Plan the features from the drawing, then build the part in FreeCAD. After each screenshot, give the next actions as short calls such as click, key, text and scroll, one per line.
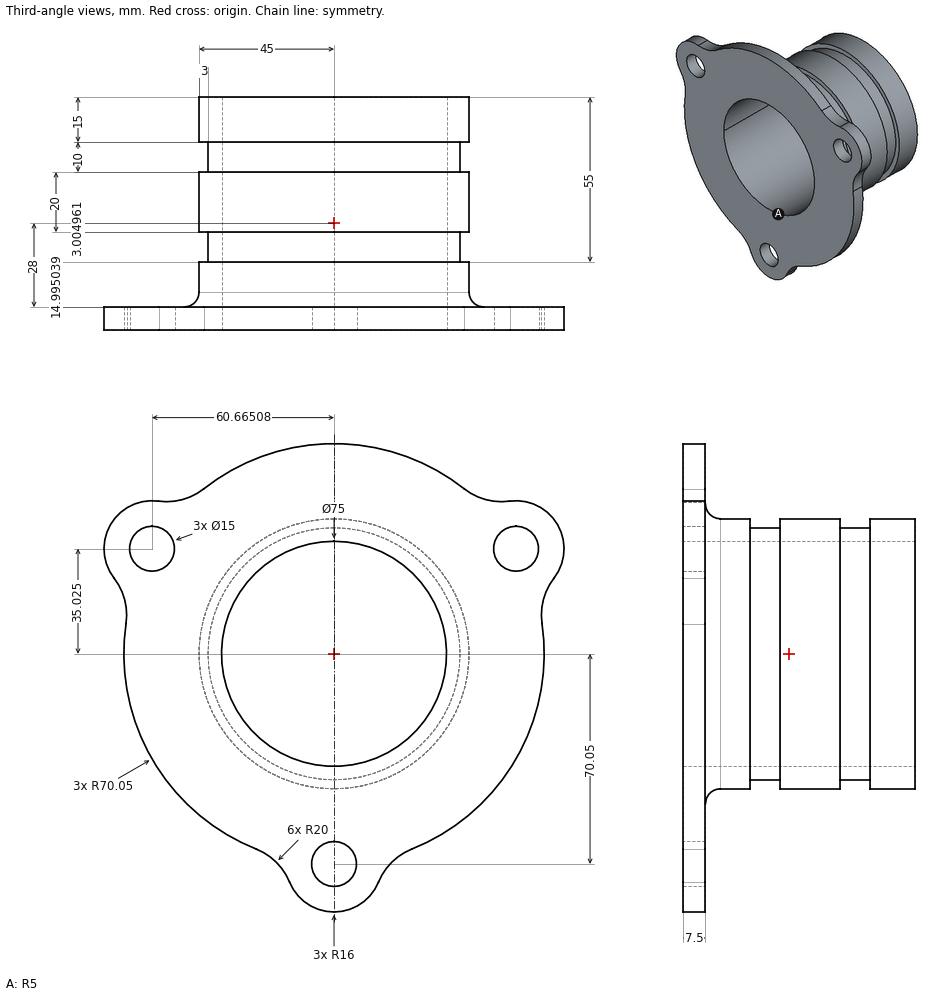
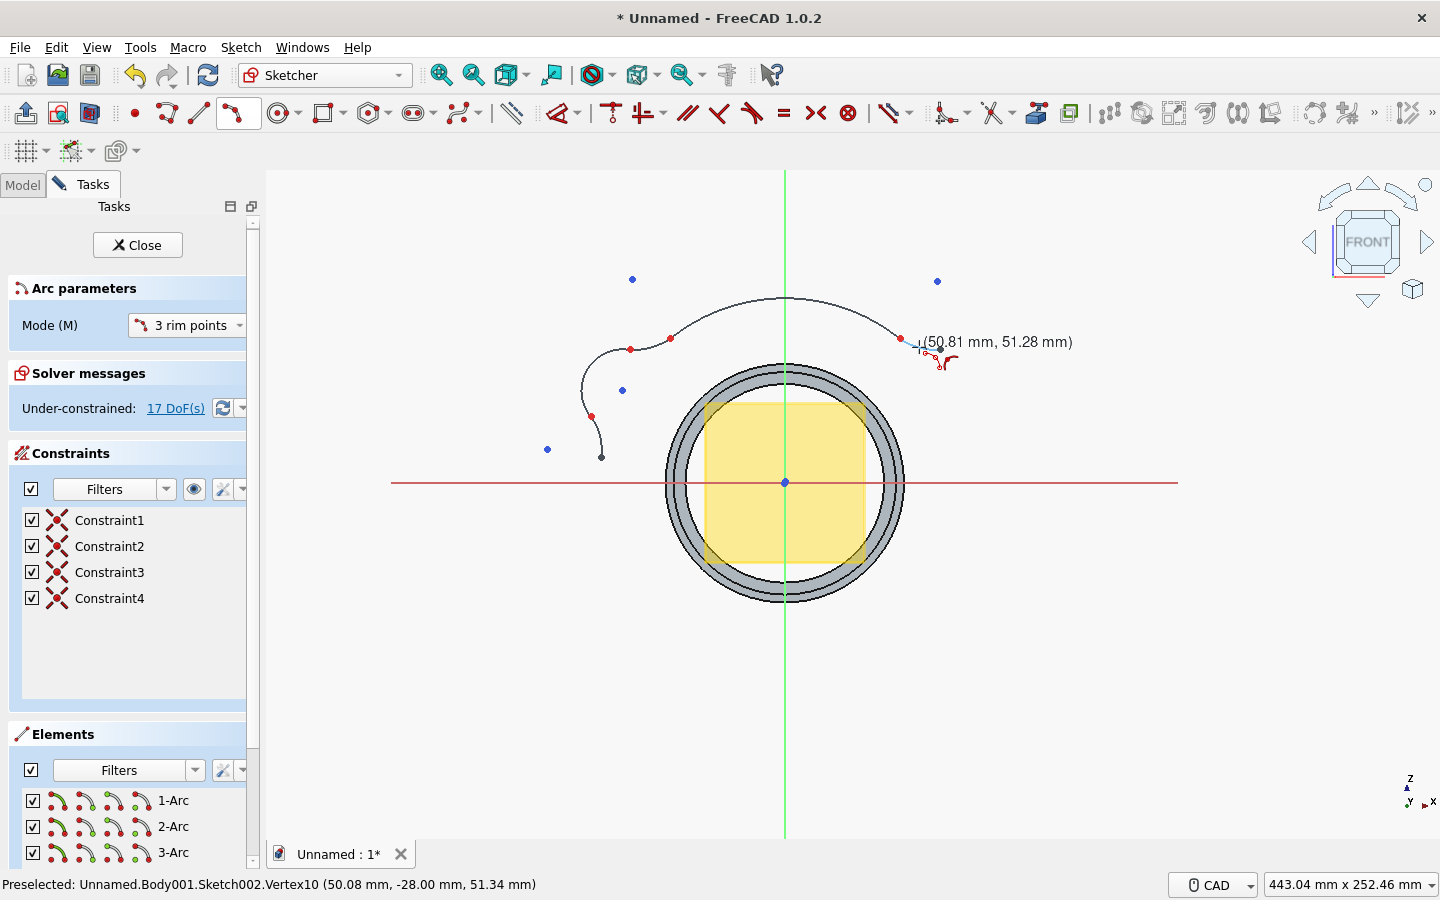
click(940, 350)
click(979, 416)
click(982, 369)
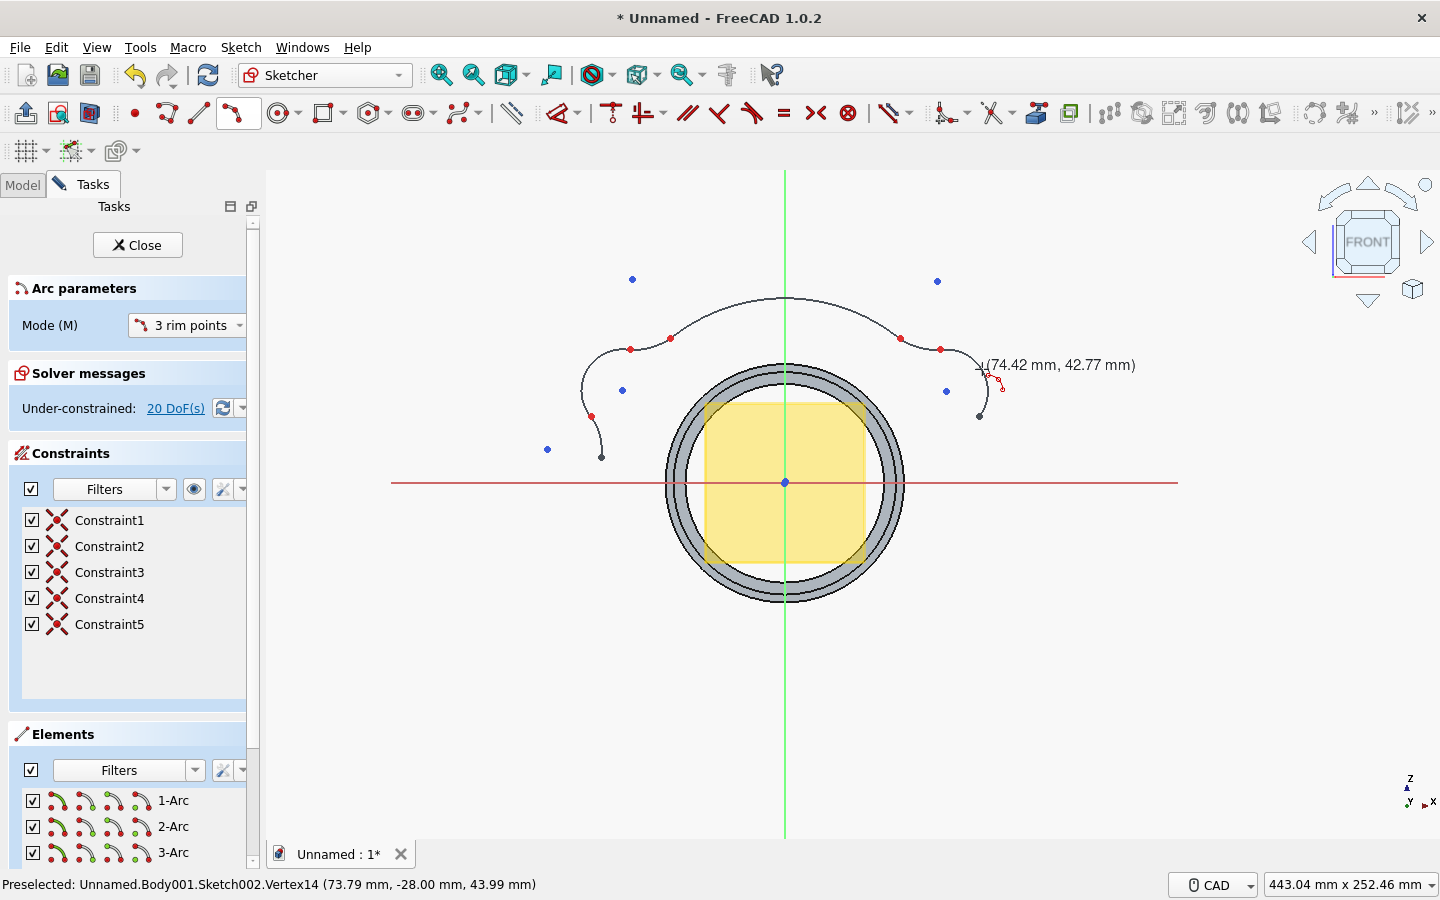
click(979, 417)
click(968, 457)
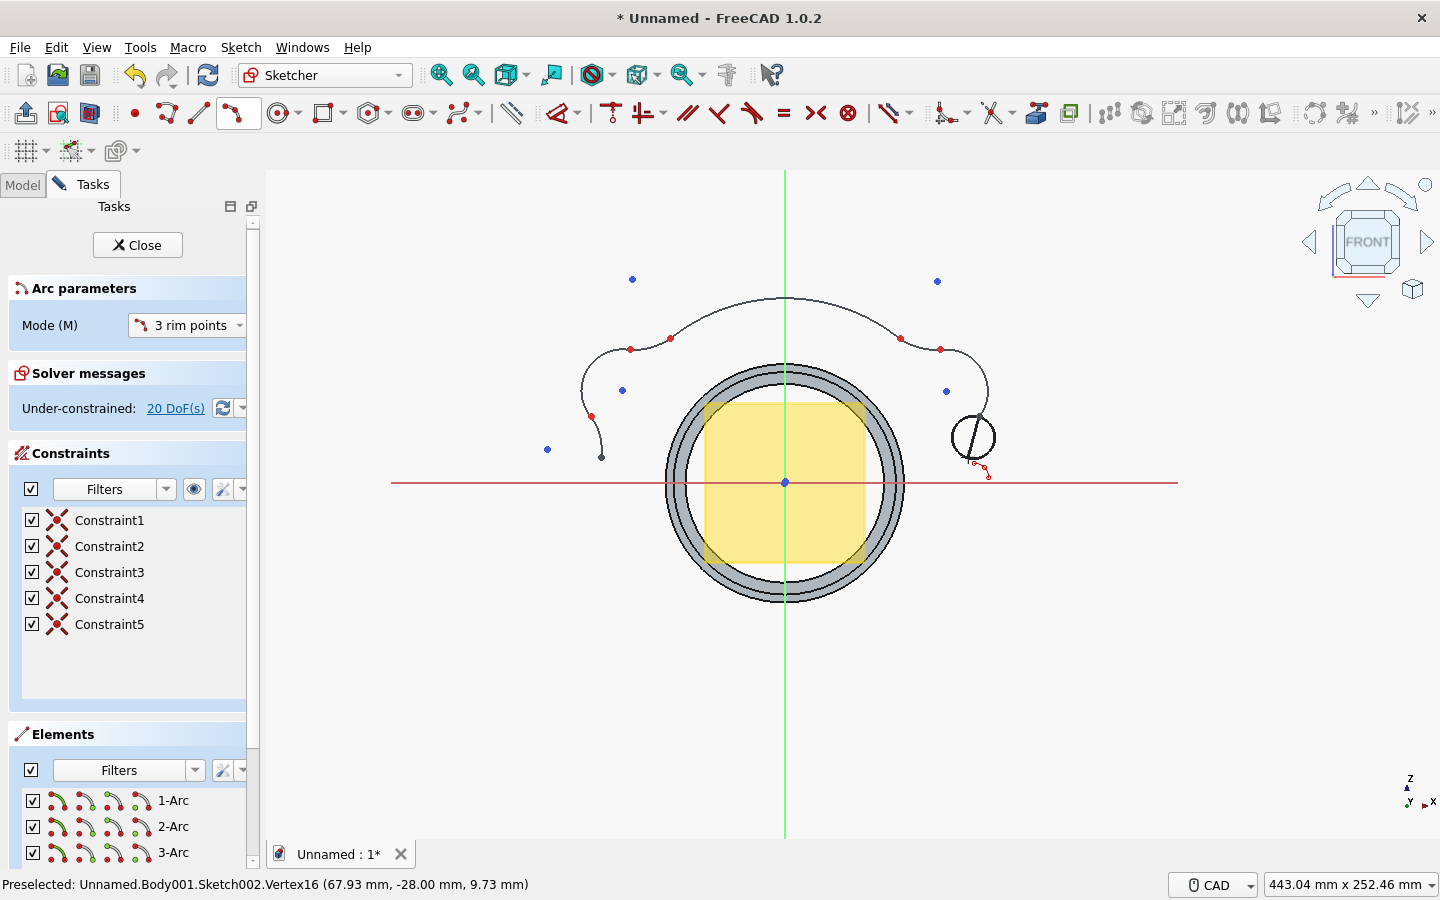
scroll(970, 435, up, 7)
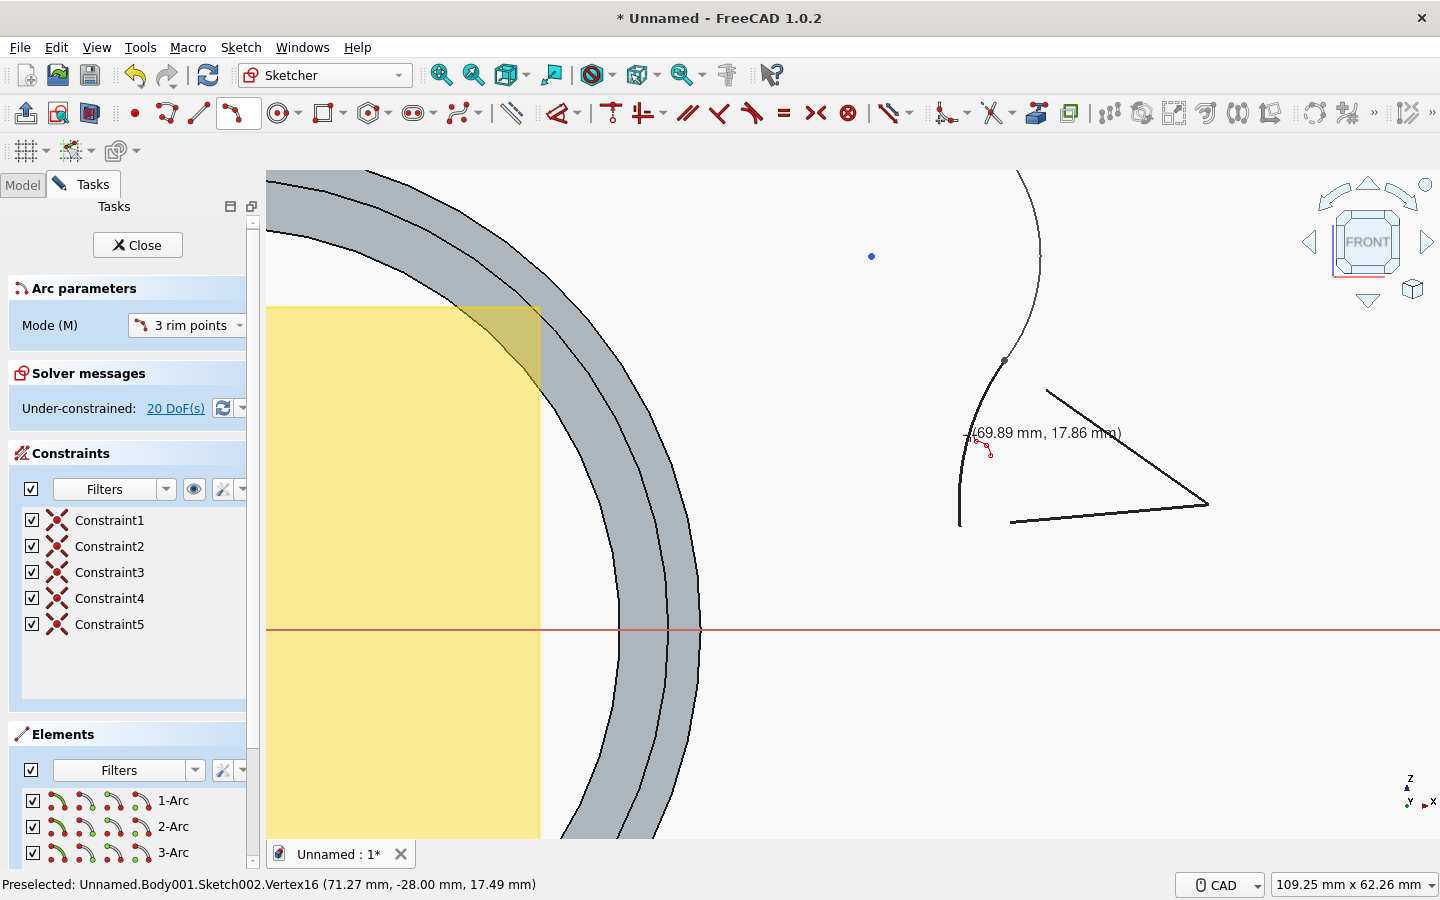
click(967, 436)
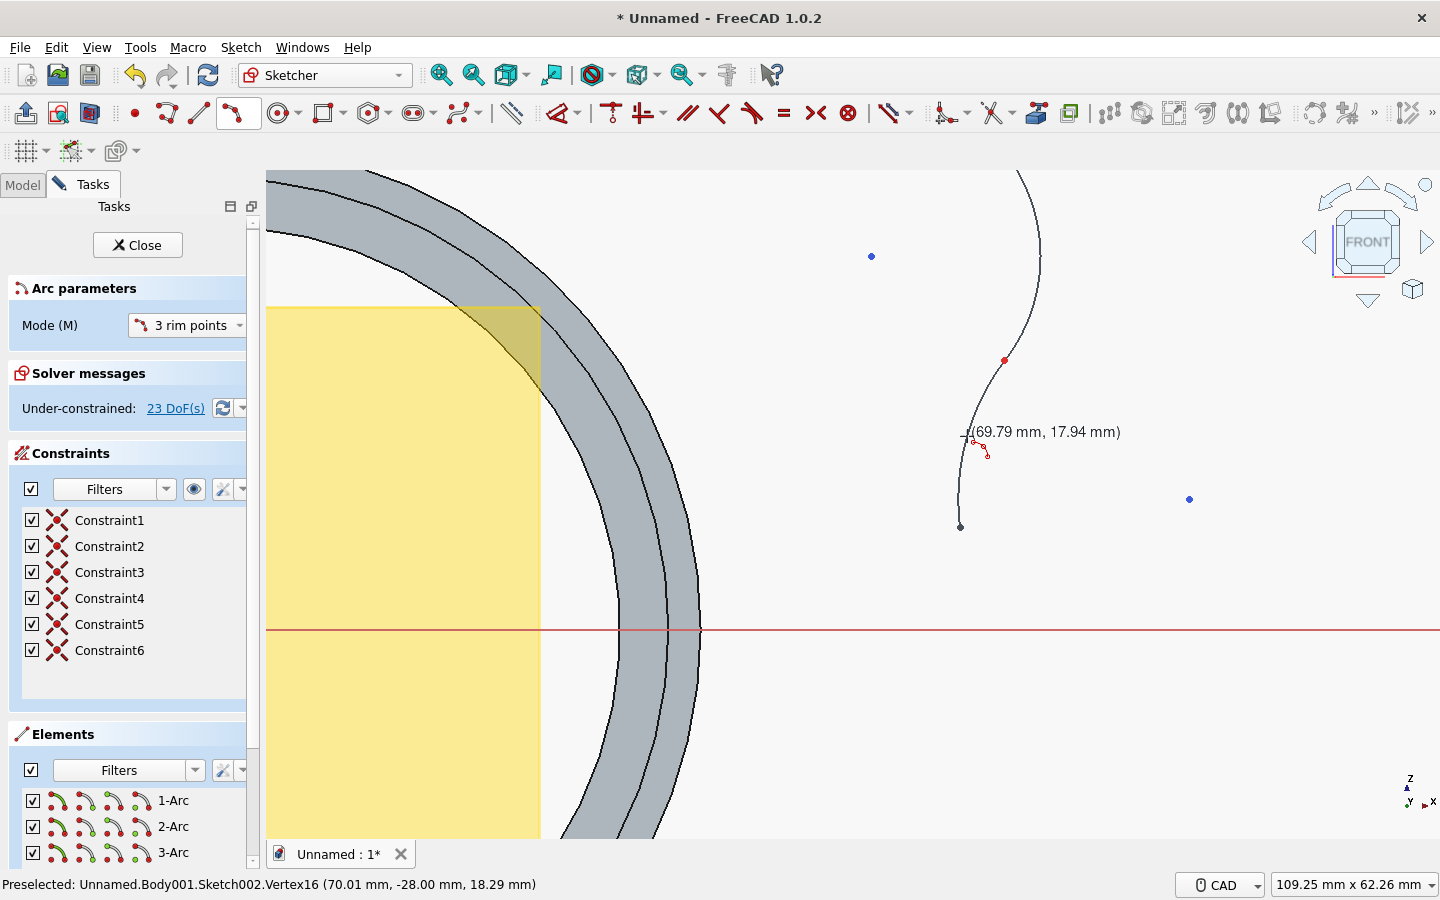
scroll(970, 435, down, 7)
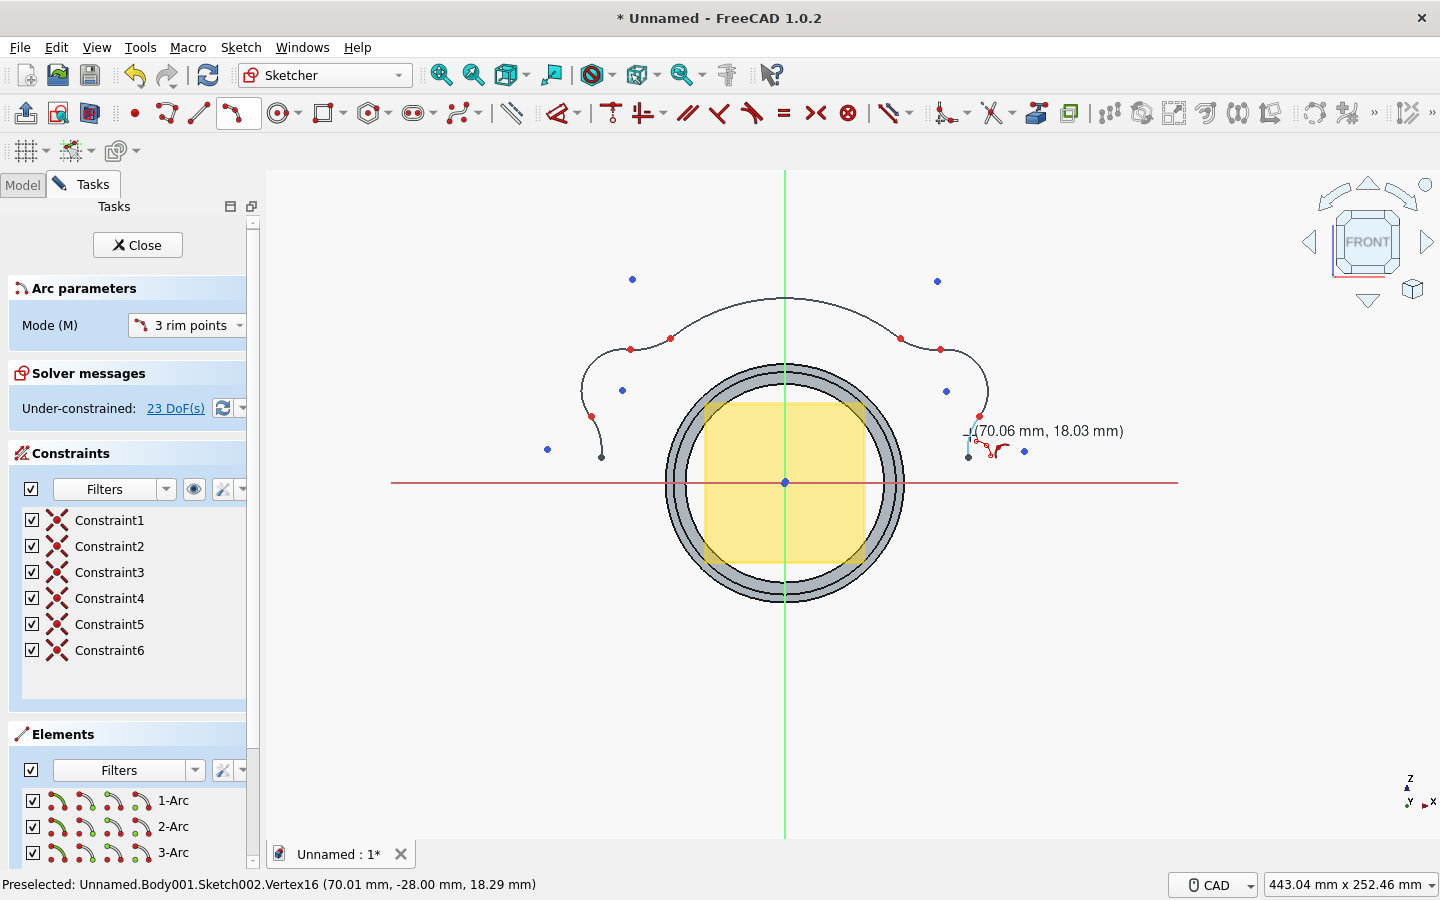
click(968, 458)
click(853, 656)
click(946, 576)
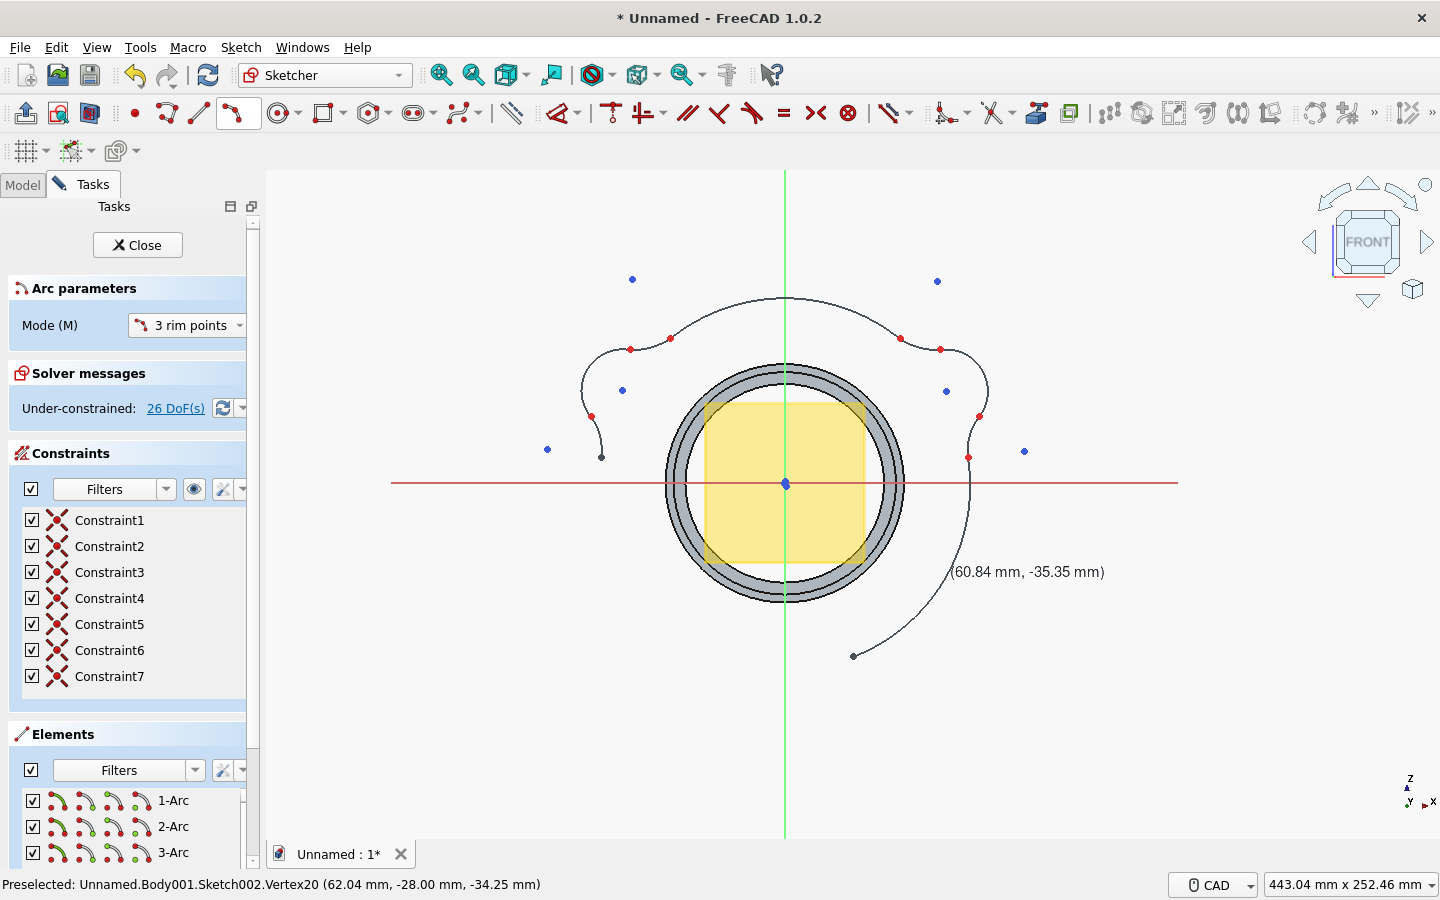
click(853, 657)
click(824, 685)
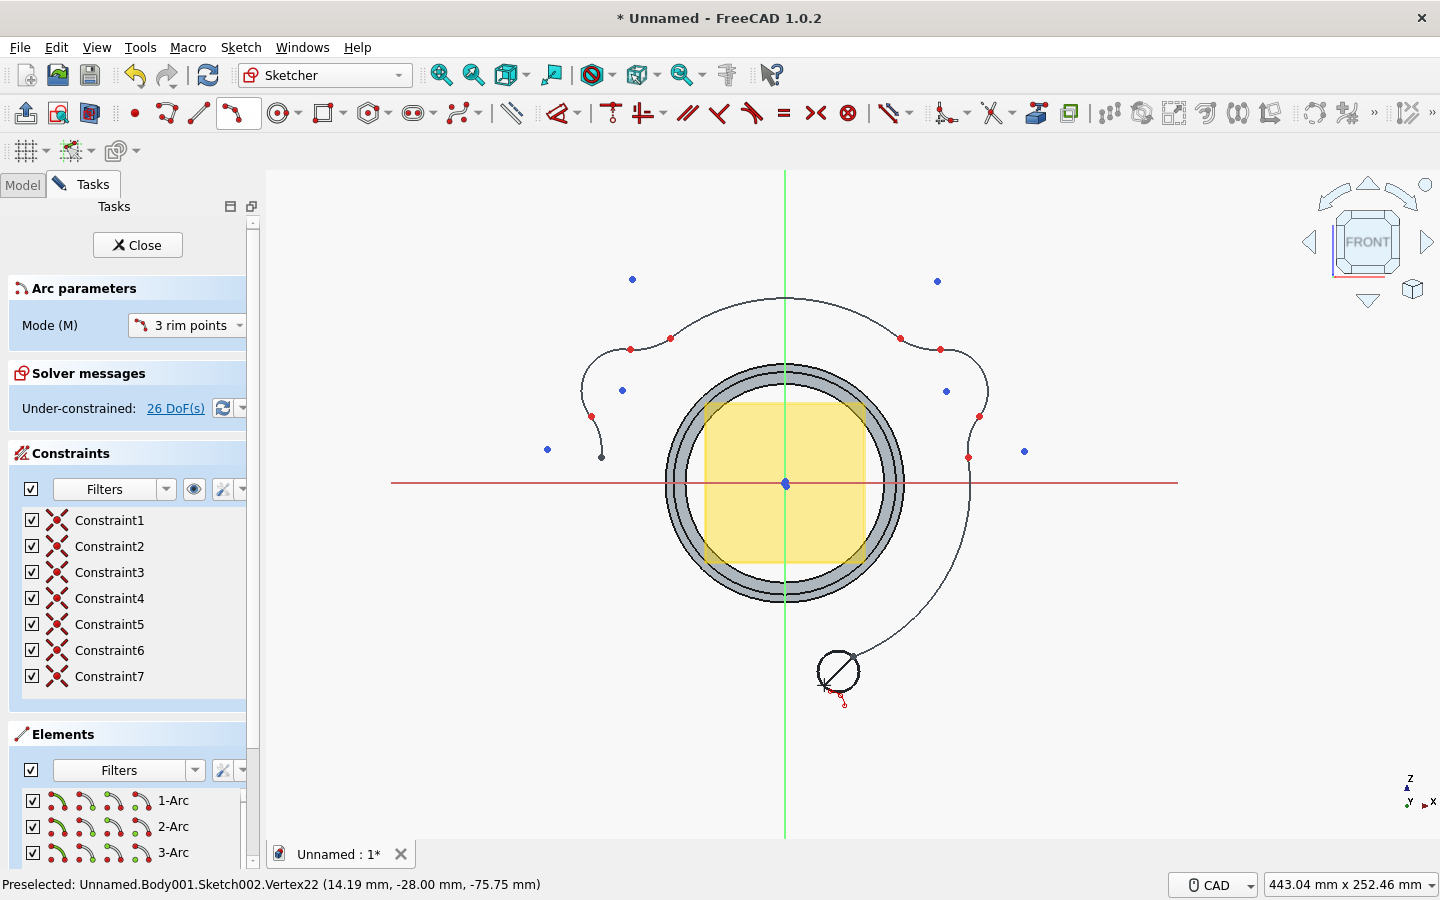
scroll(836, 667, up, 7)